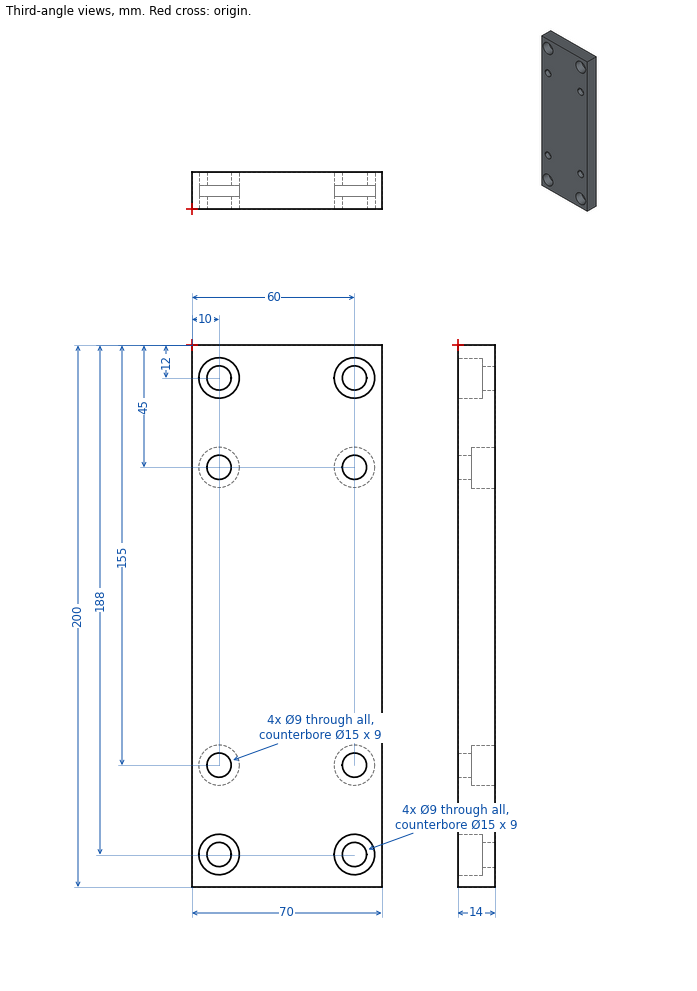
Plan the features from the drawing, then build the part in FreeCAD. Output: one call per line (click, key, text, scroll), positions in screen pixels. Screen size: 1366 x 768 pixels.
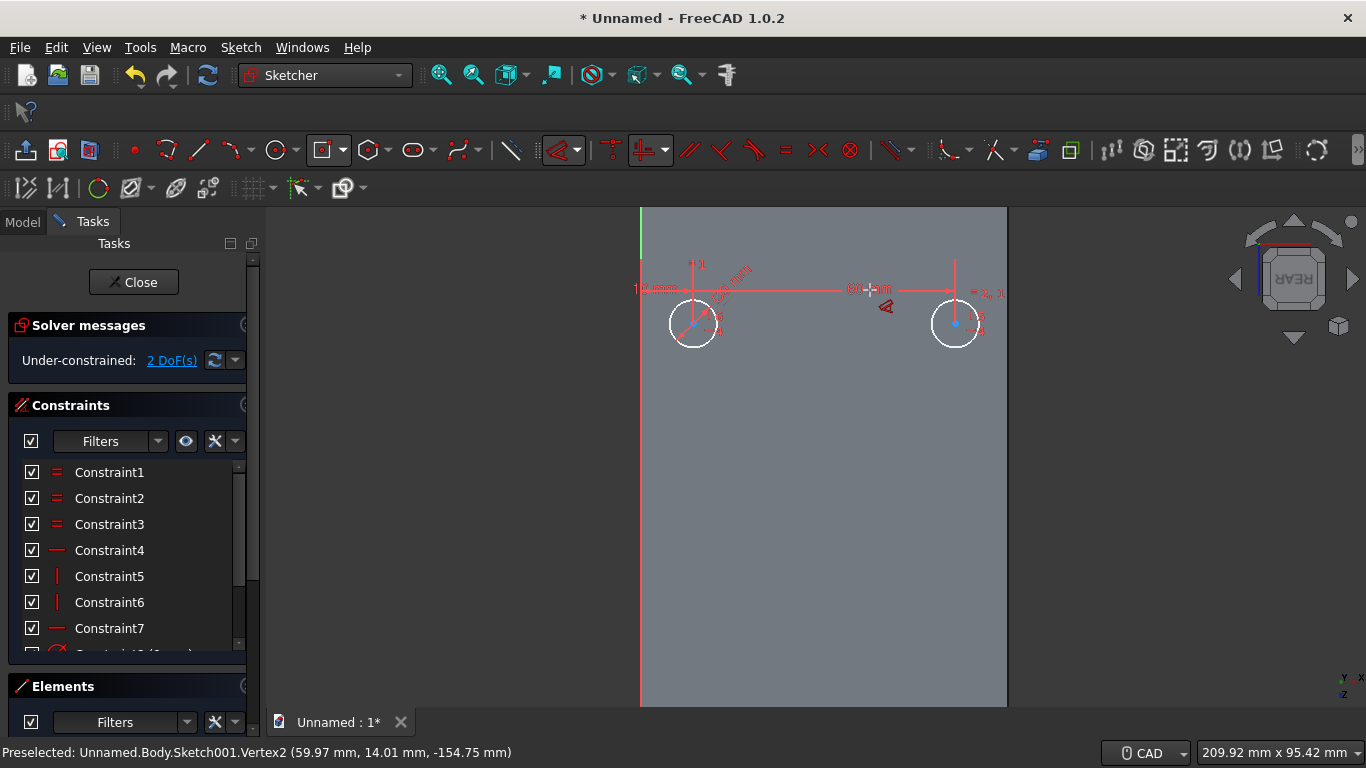
scroll(711, 306, down, 5)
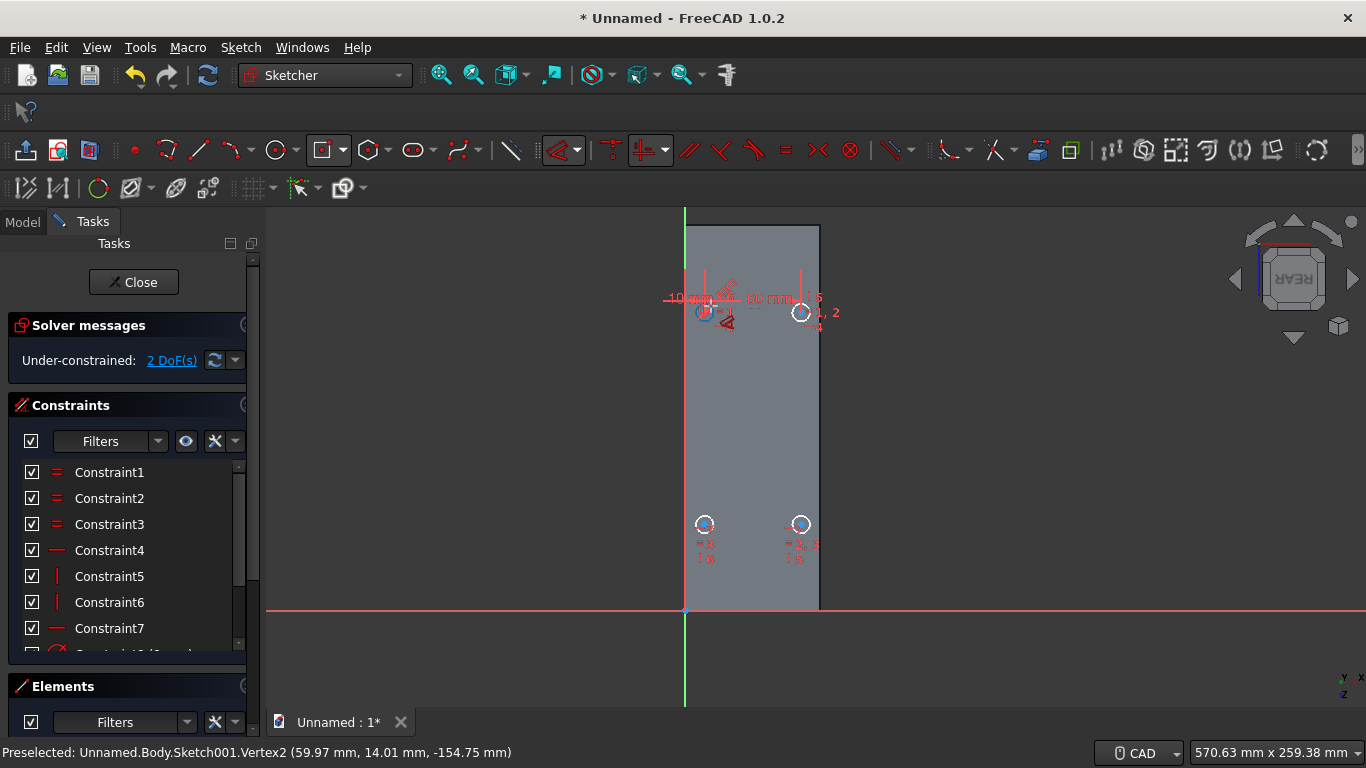
click(801, 525)
click(651, 568)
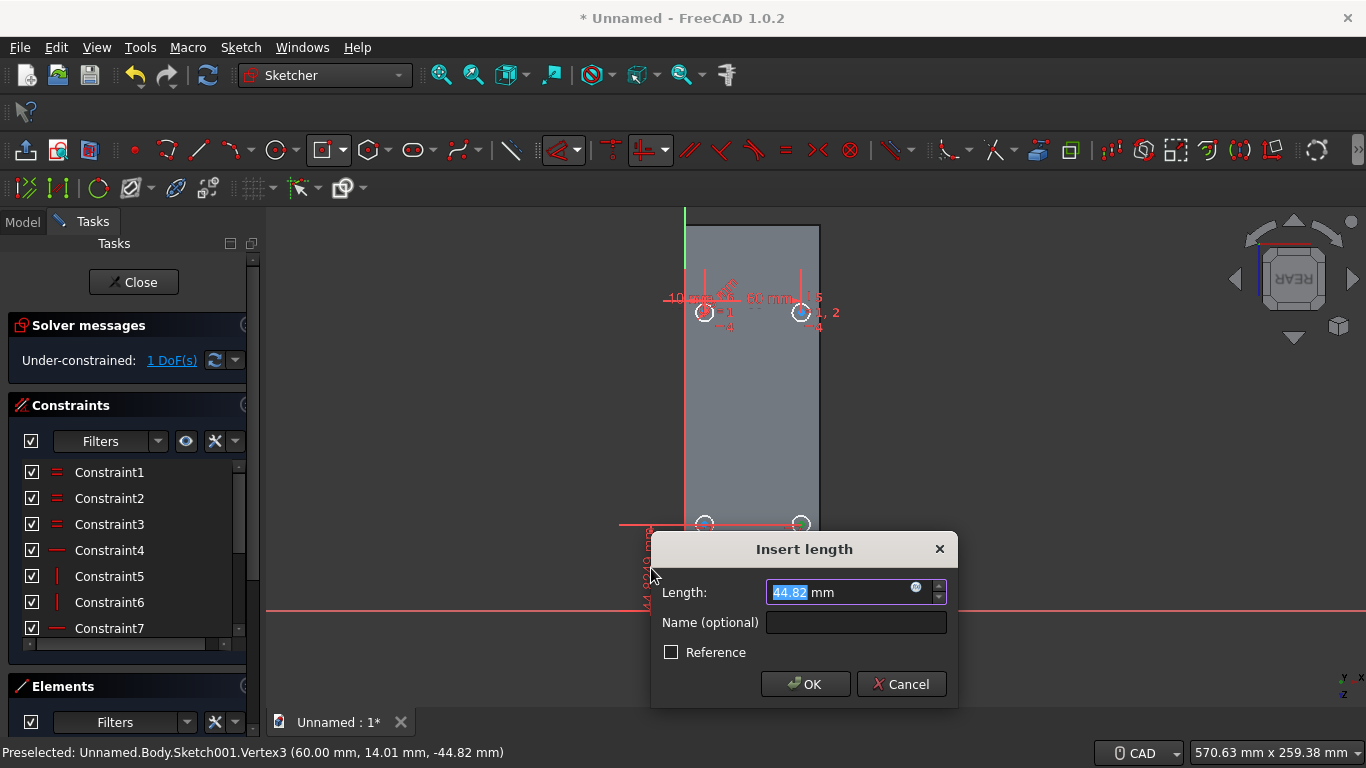
text(45)
key(Return)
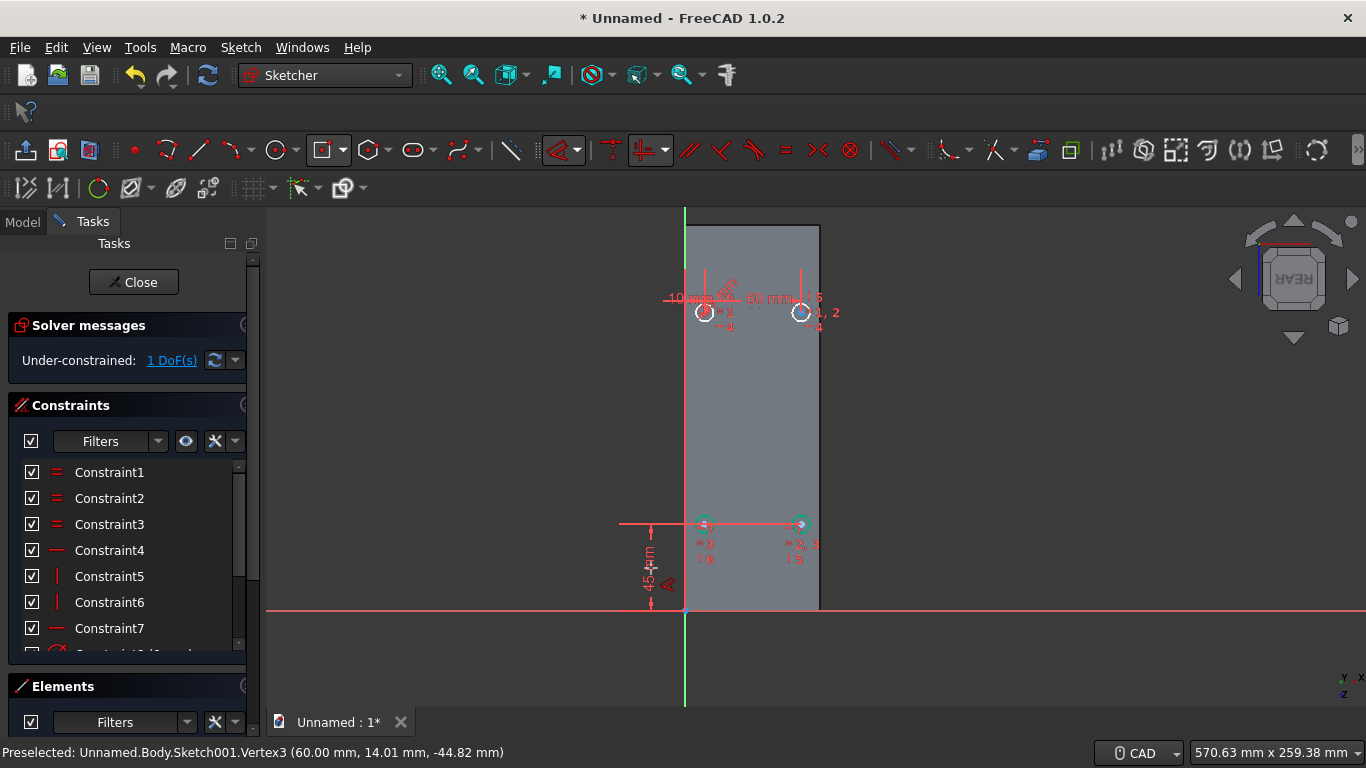
click(705, 313)
click(651, 462)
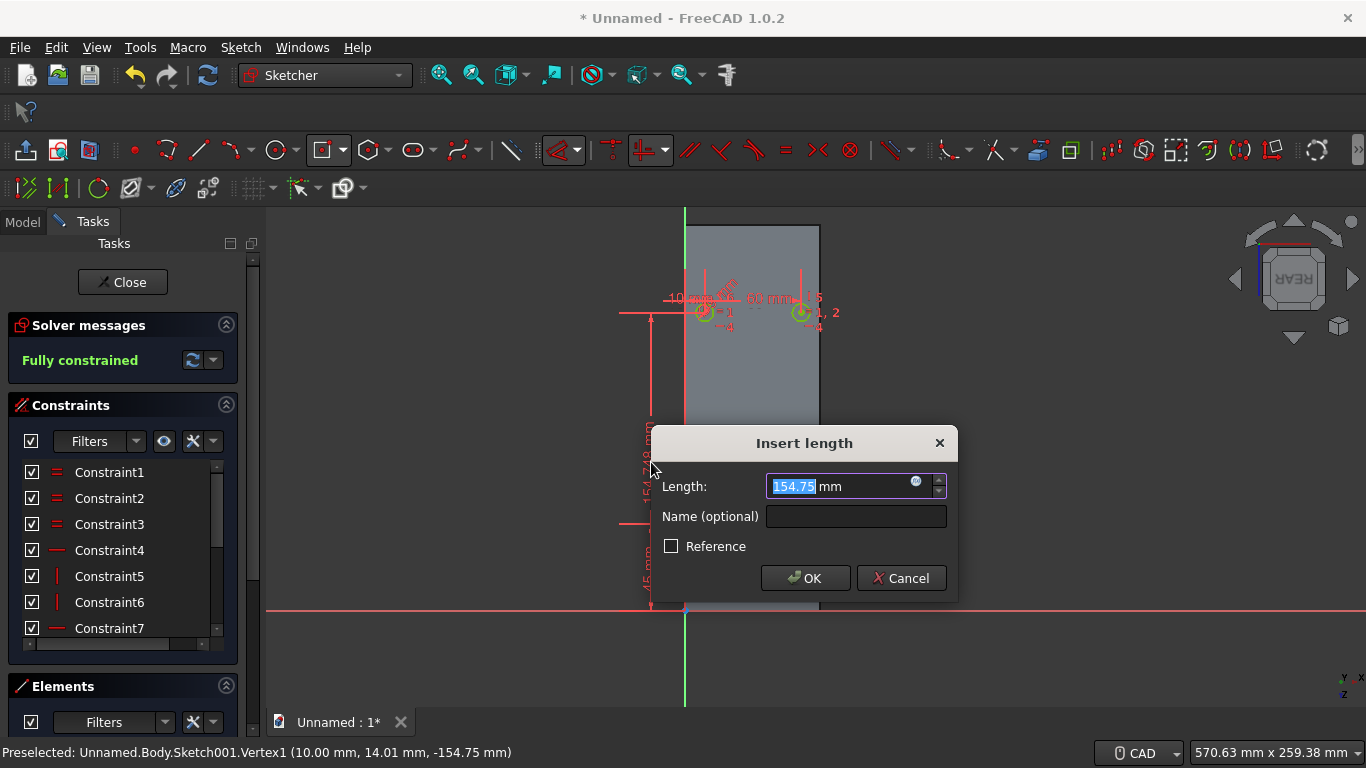
text(155)
key(Return)
key(Escape)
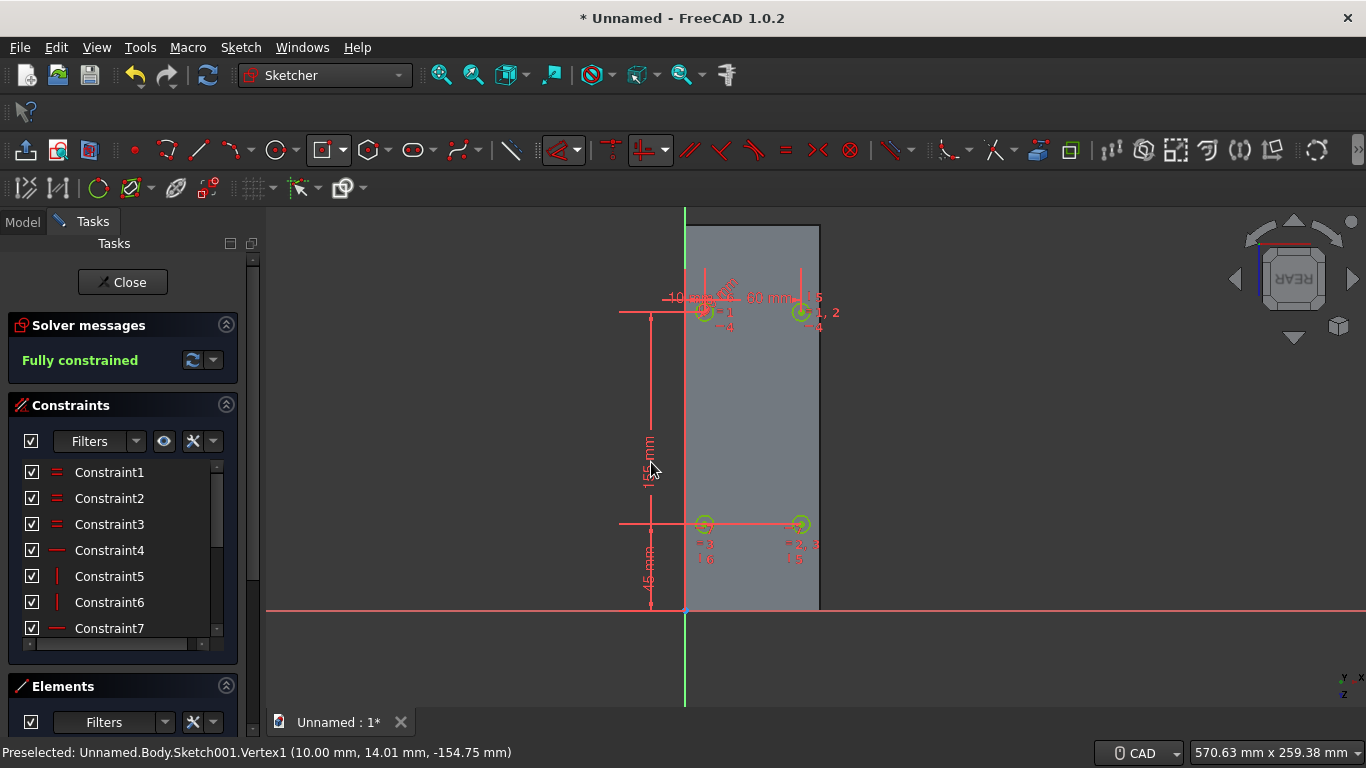
click(123, 282)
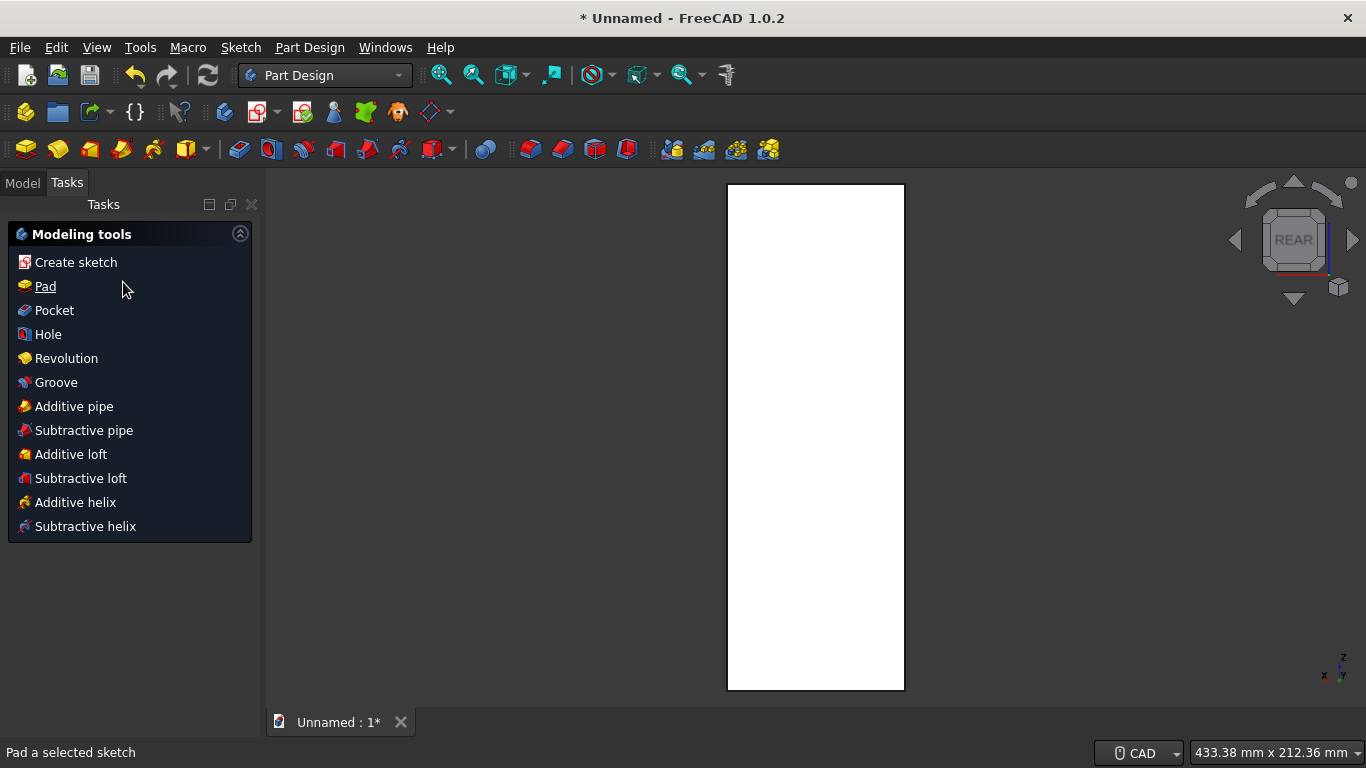
click(272, 150)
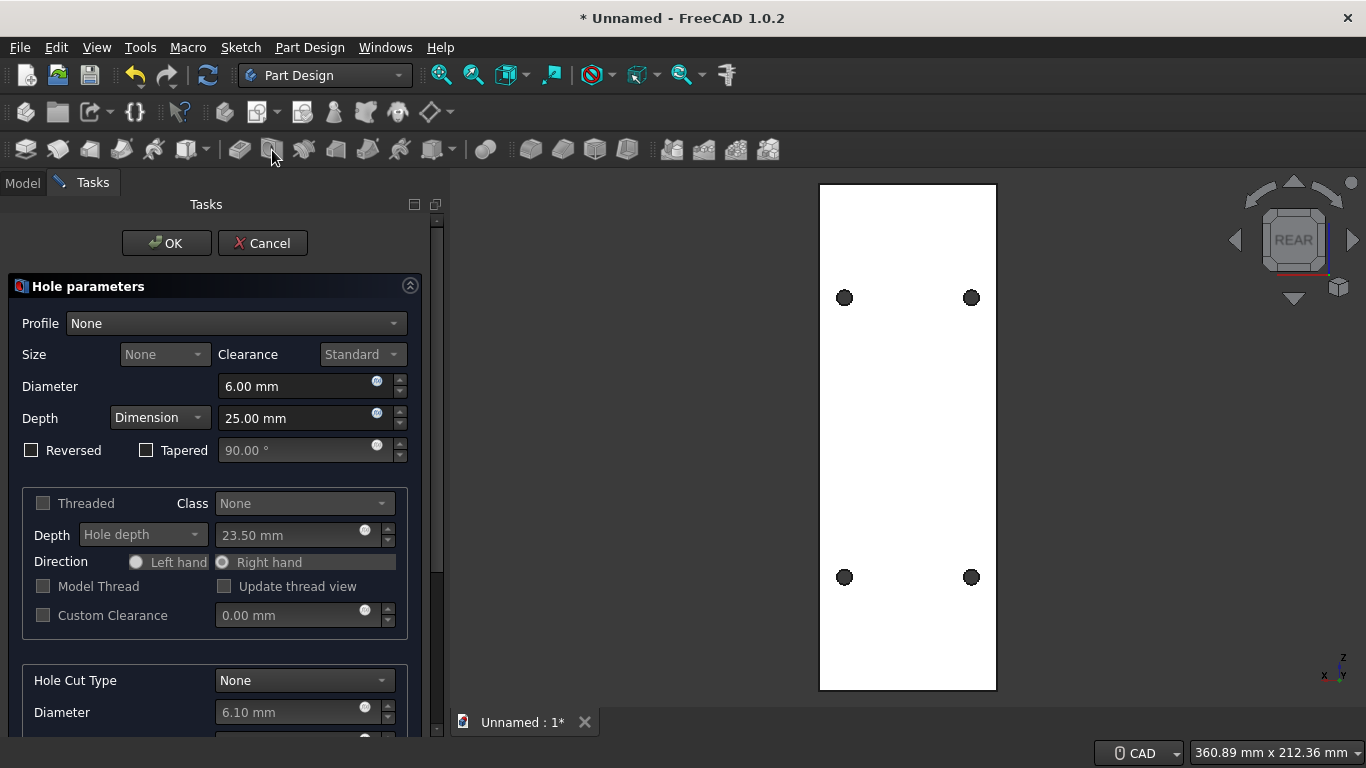
triple_click(305, 386)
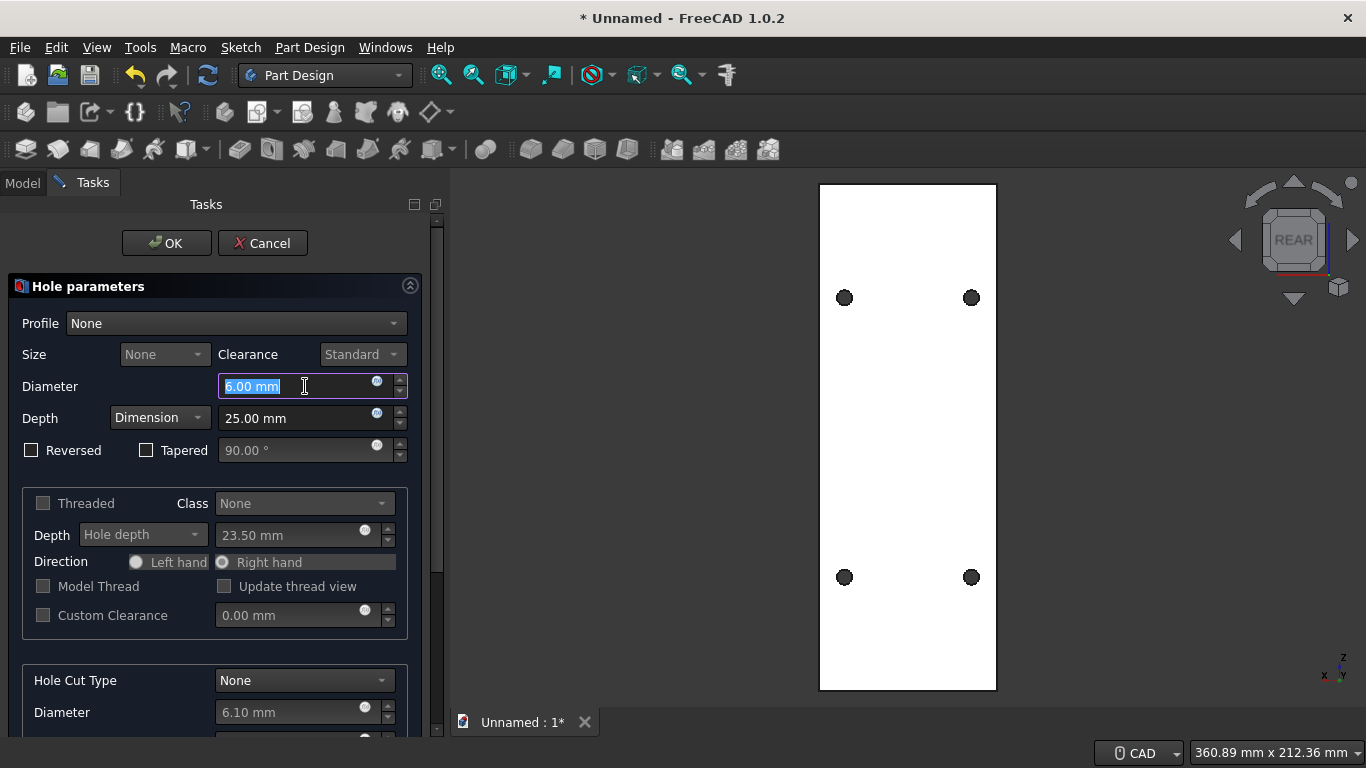
text(9)
key(Tab)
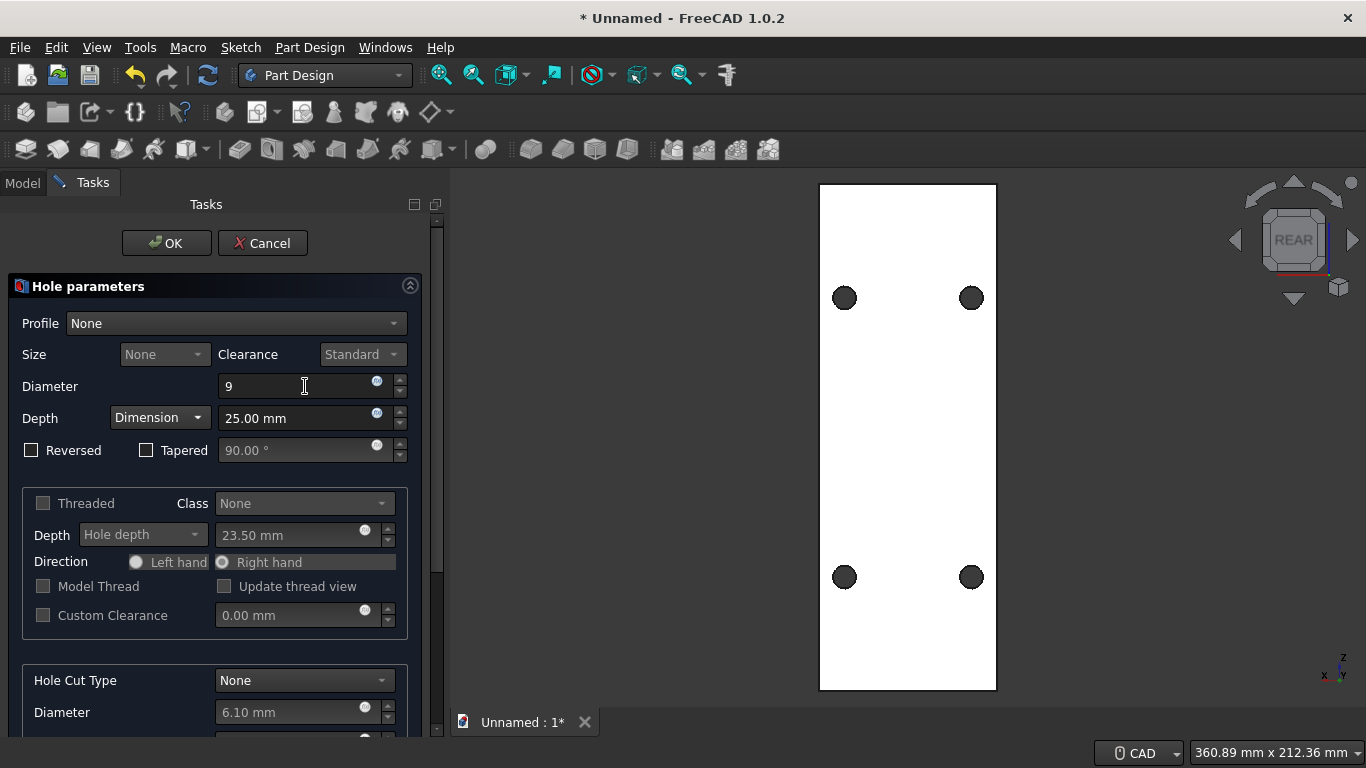
click(161, 418)